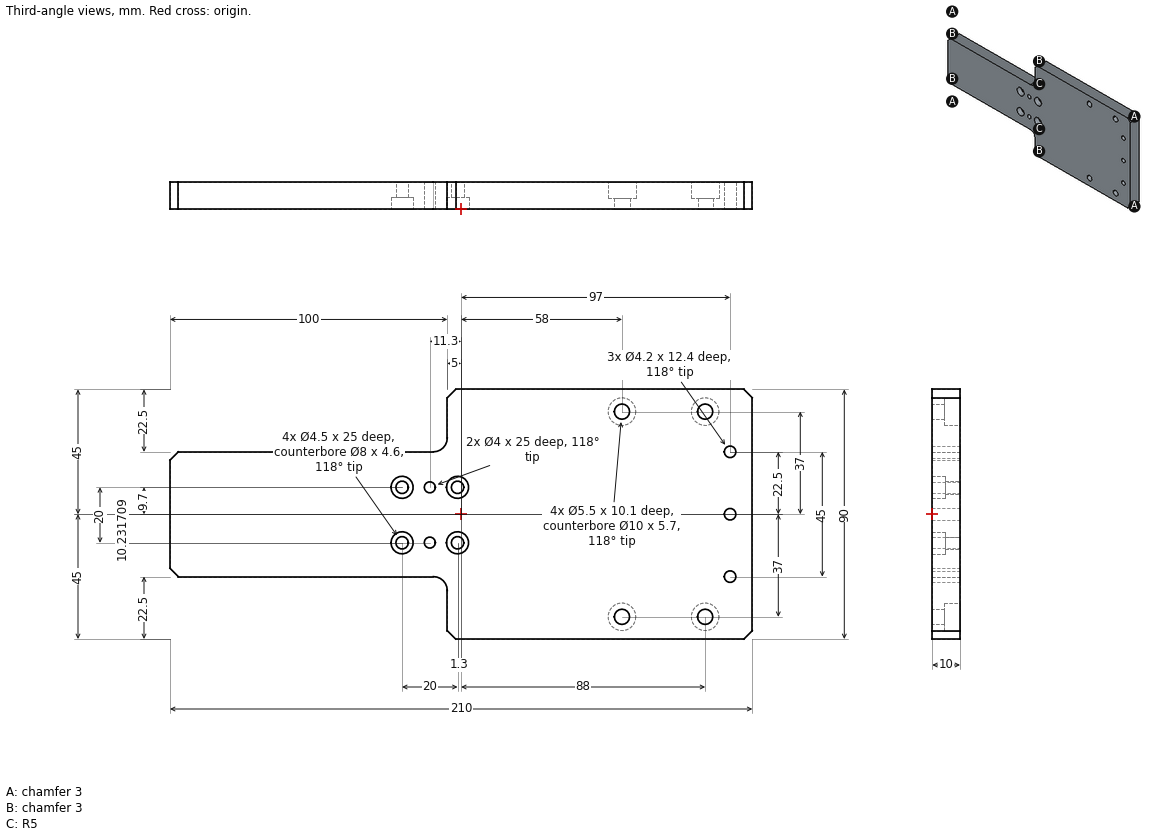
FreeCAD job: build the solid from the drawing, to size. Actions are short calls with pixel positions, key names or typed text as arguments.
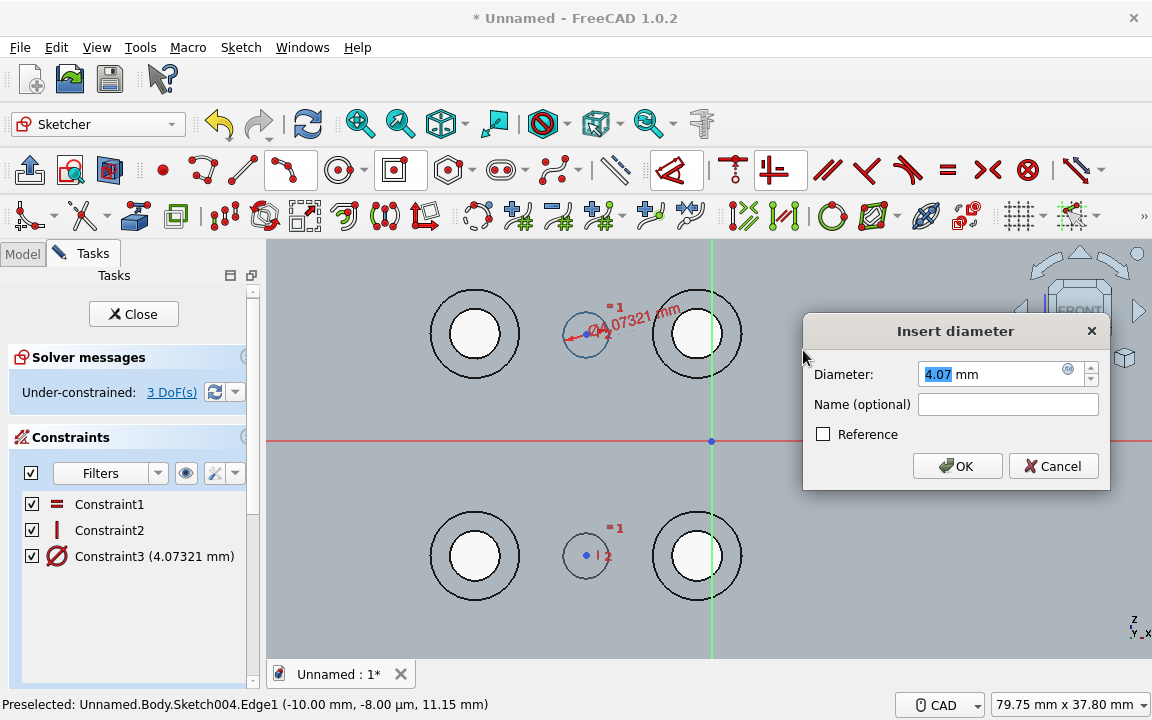
text(4)
key(Return)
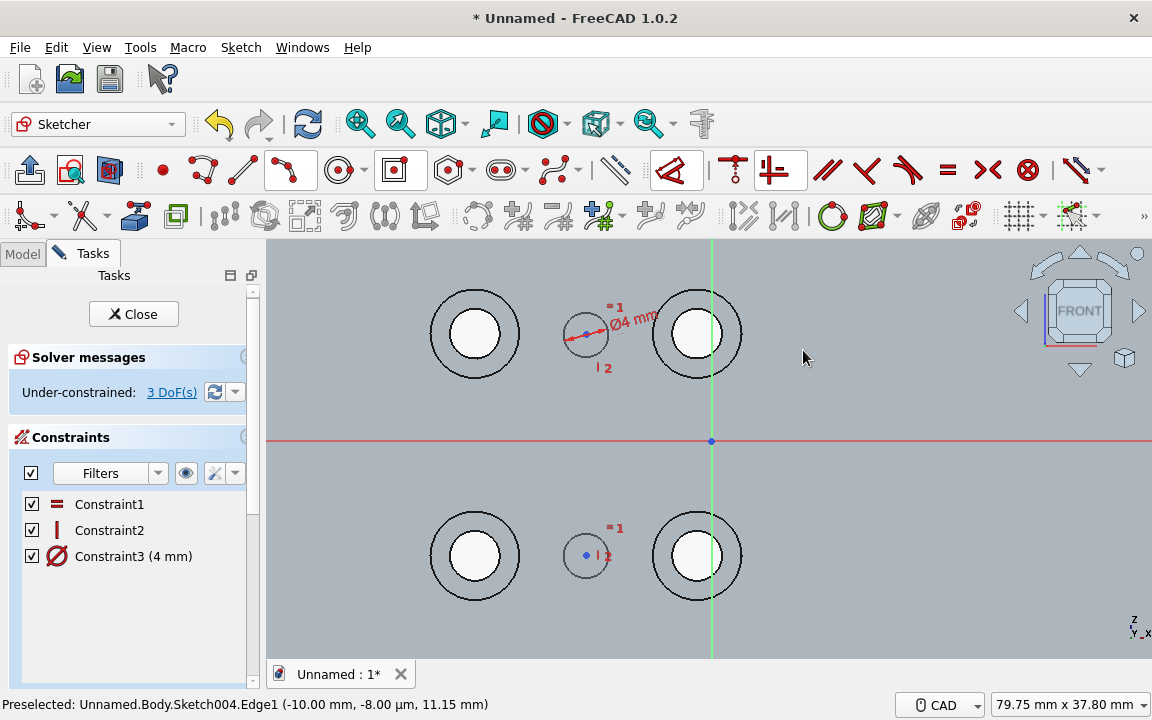
click(586, 335)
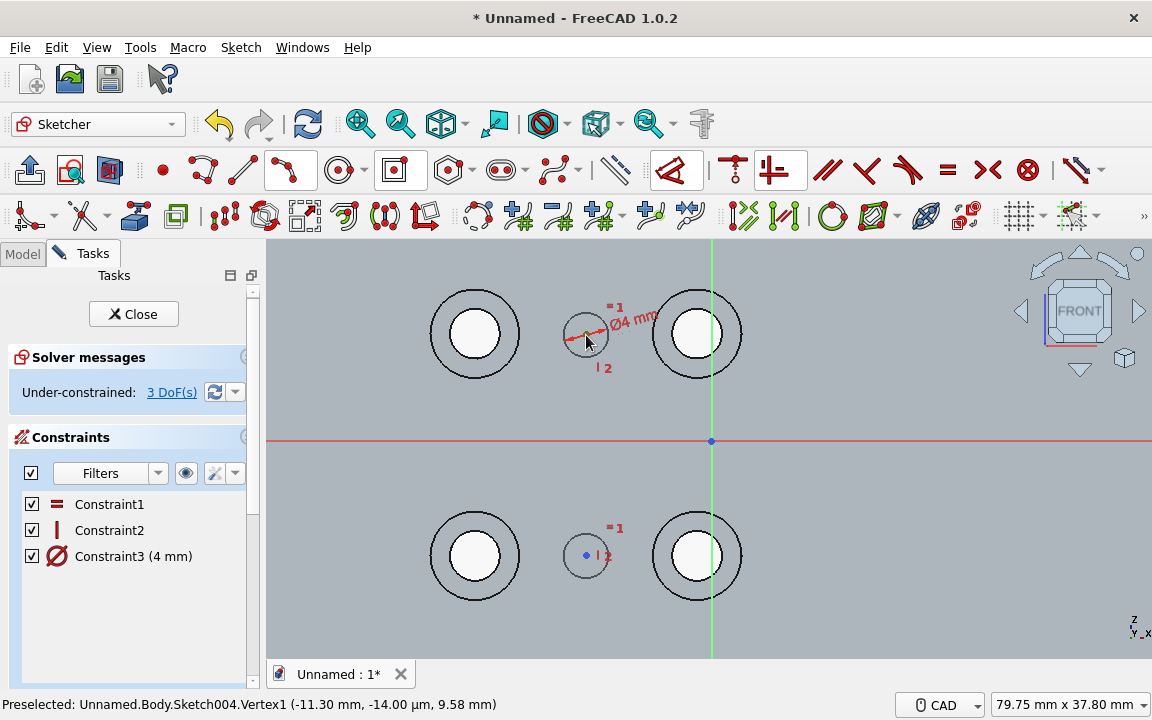
click(698, 170)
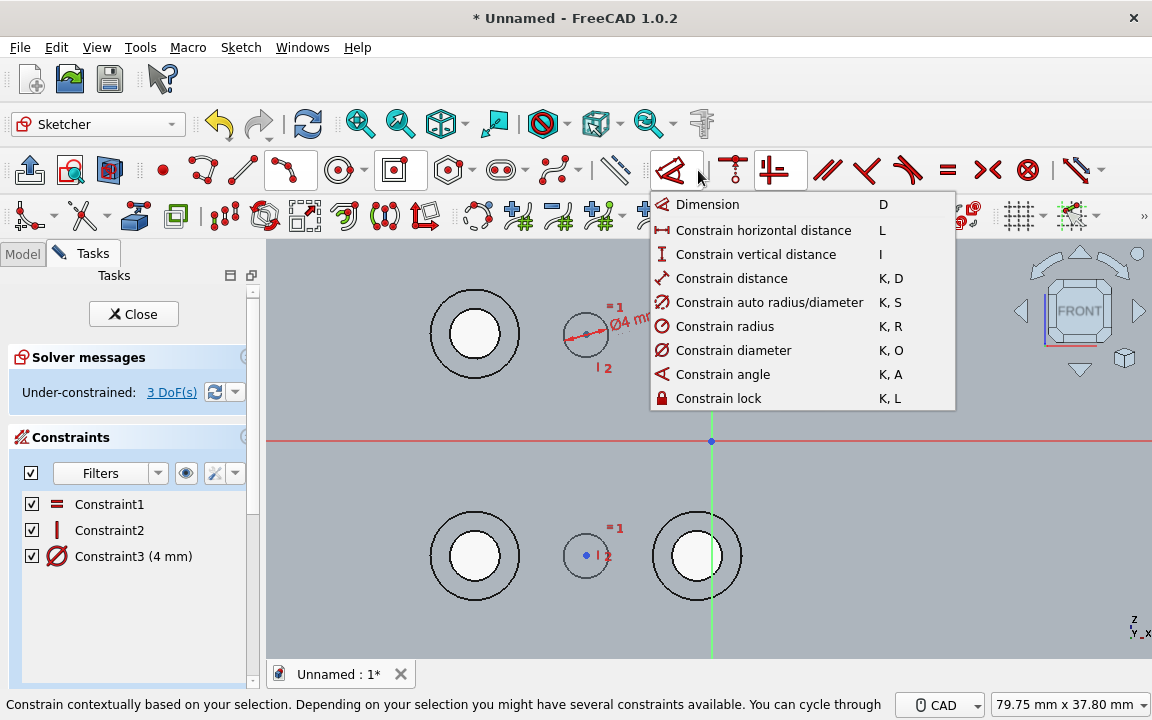
click(803, 254)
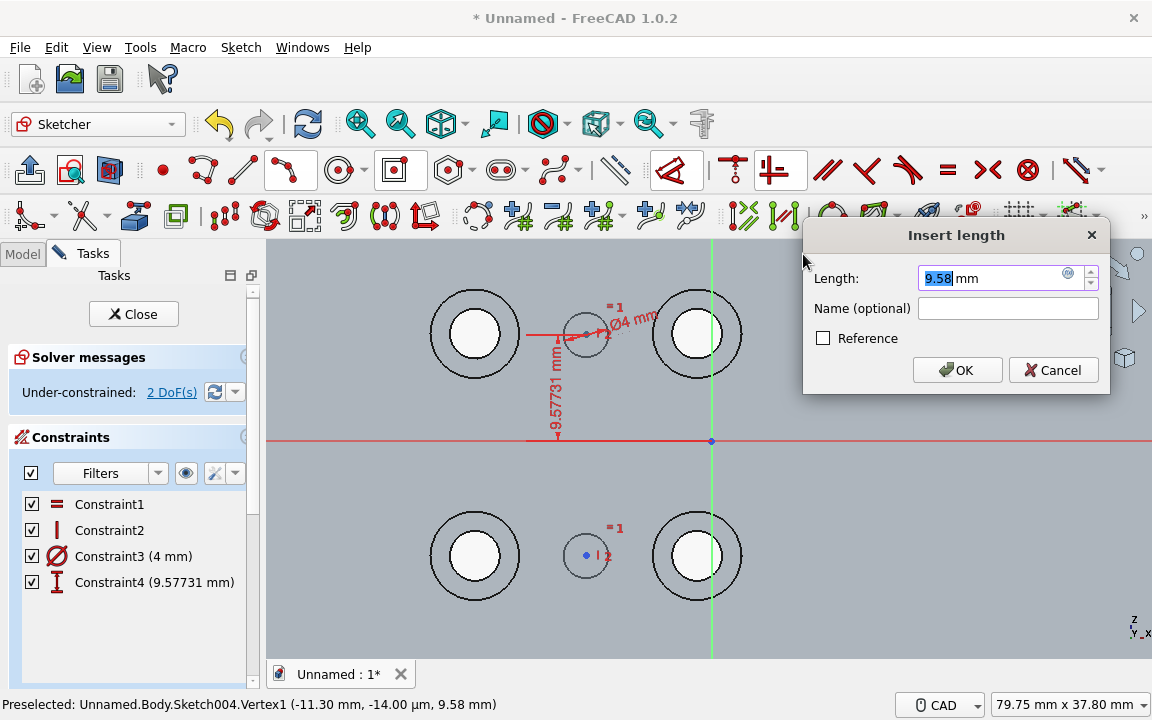
text(9.7)
key(Return)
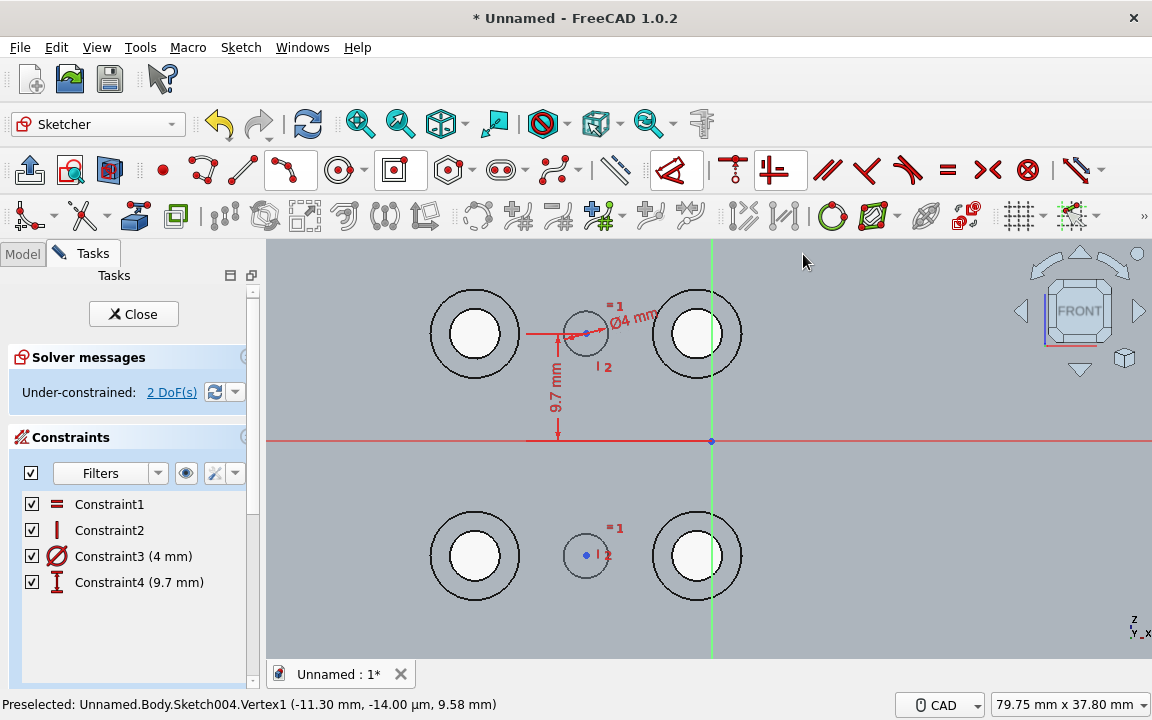
click(586, 334)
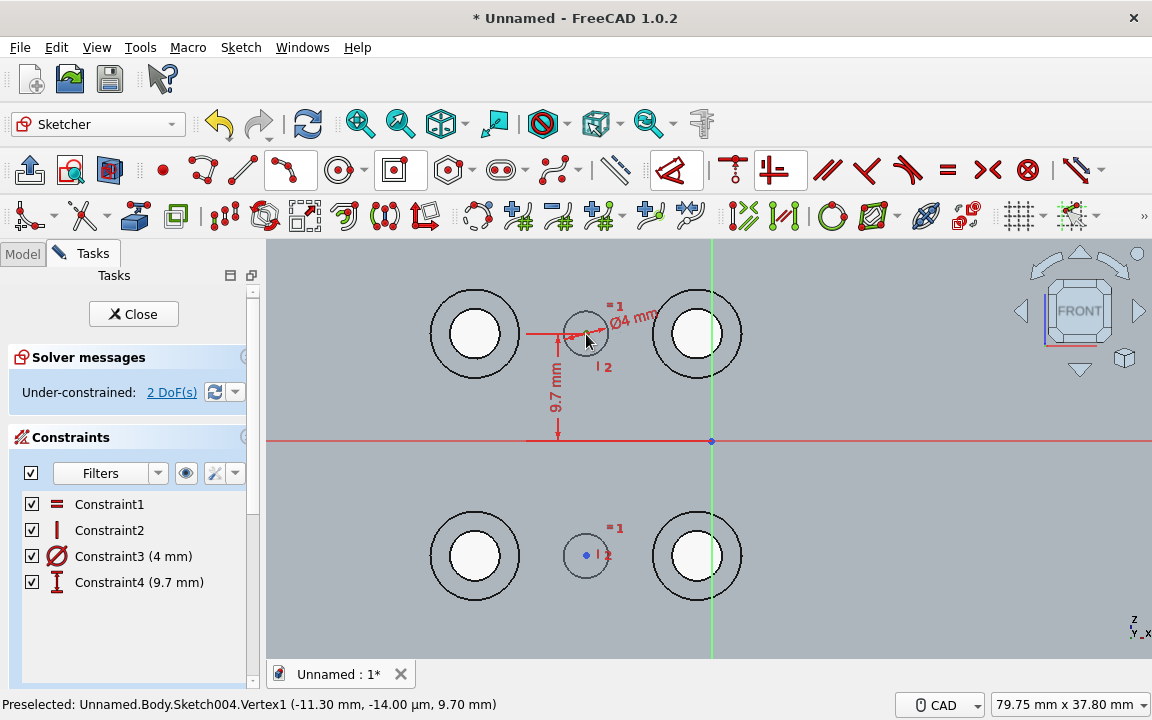
click(698, 170)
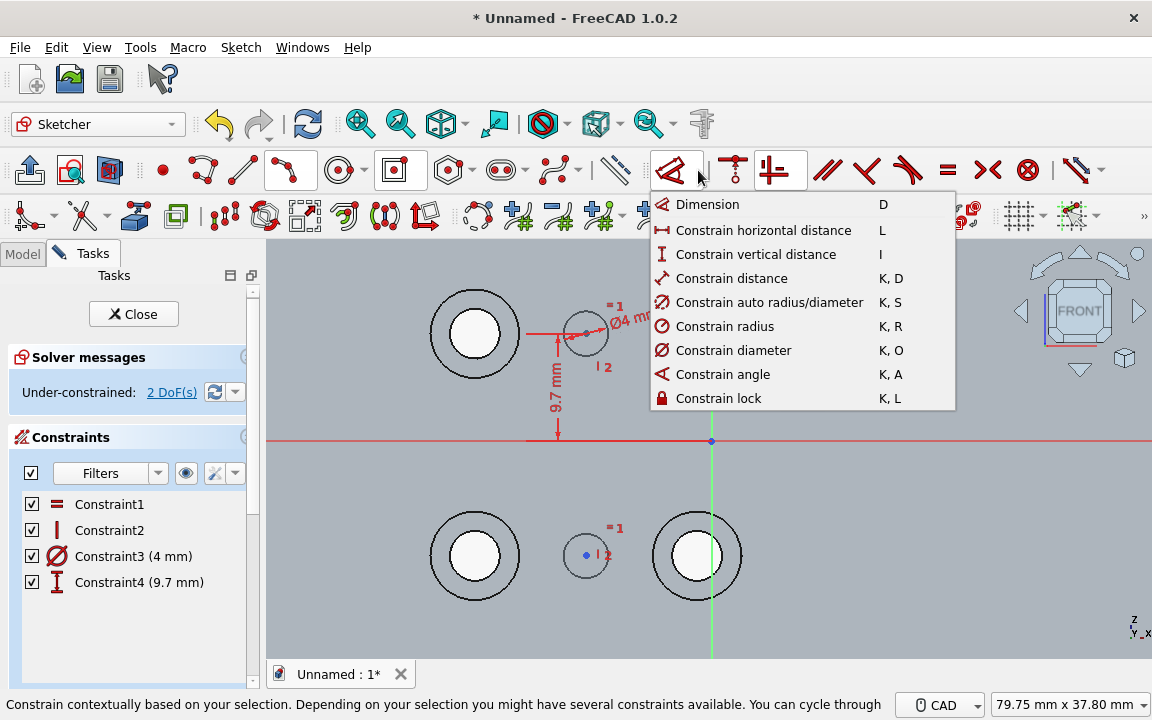
click(803, 230)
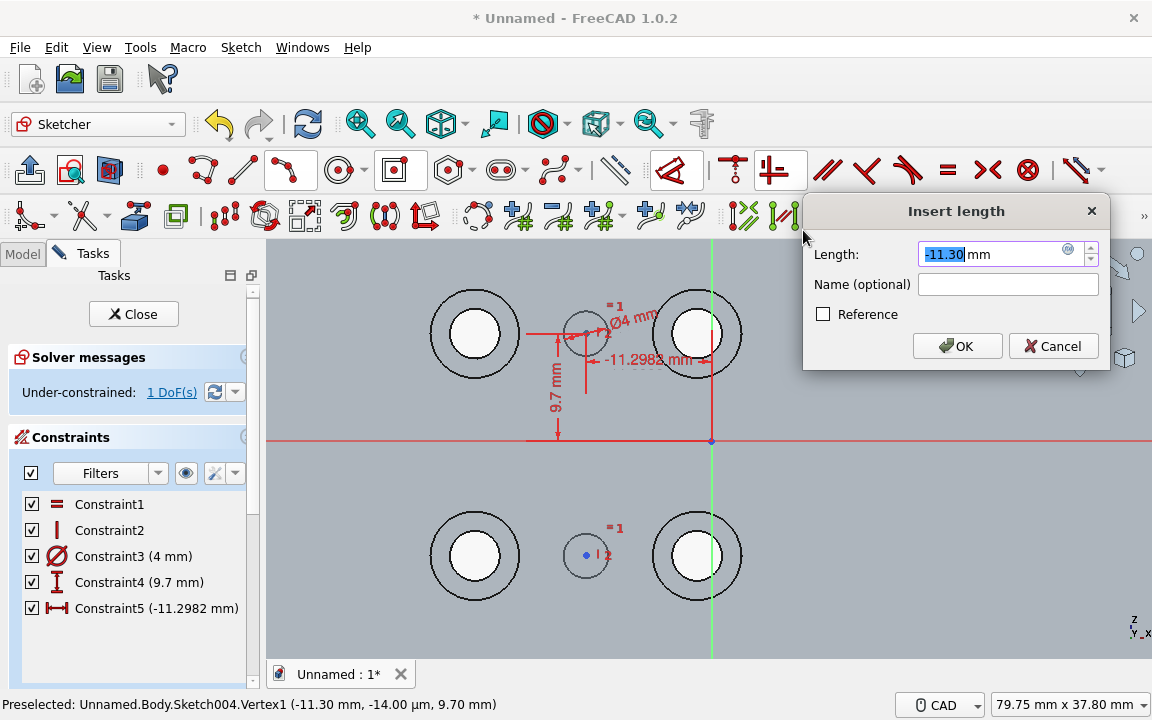
text(-11.3)
key(Return)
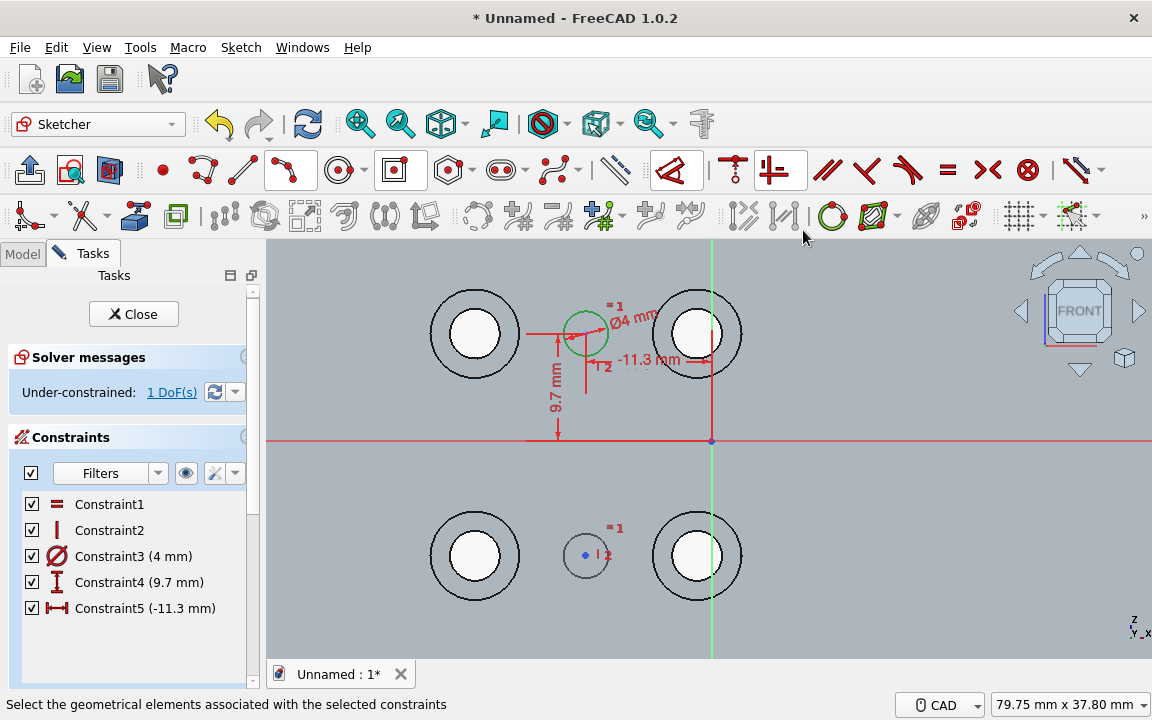
click(586, 556)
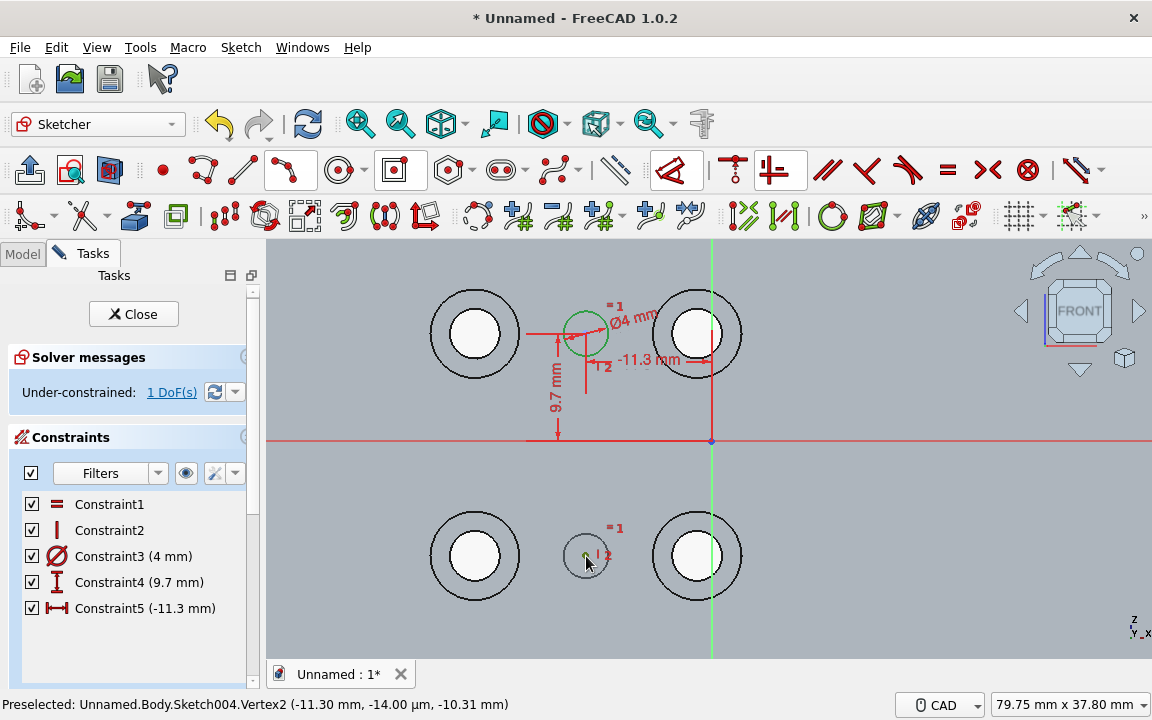
click(698, 170)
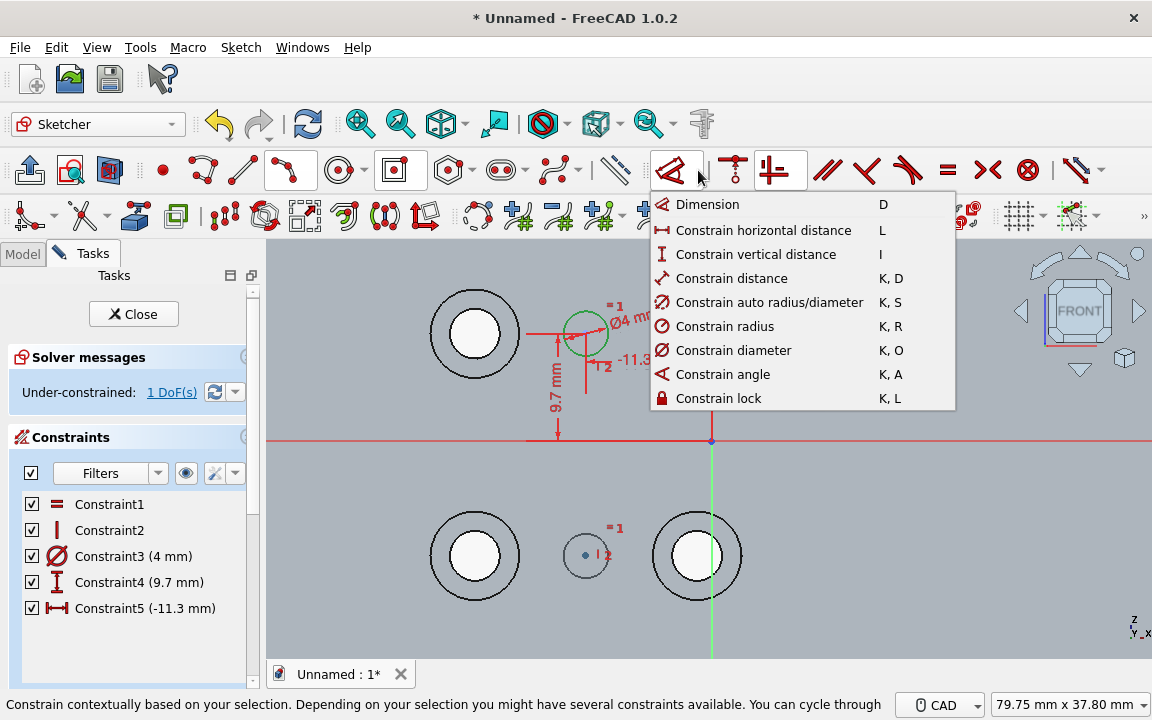
click(803, 254)